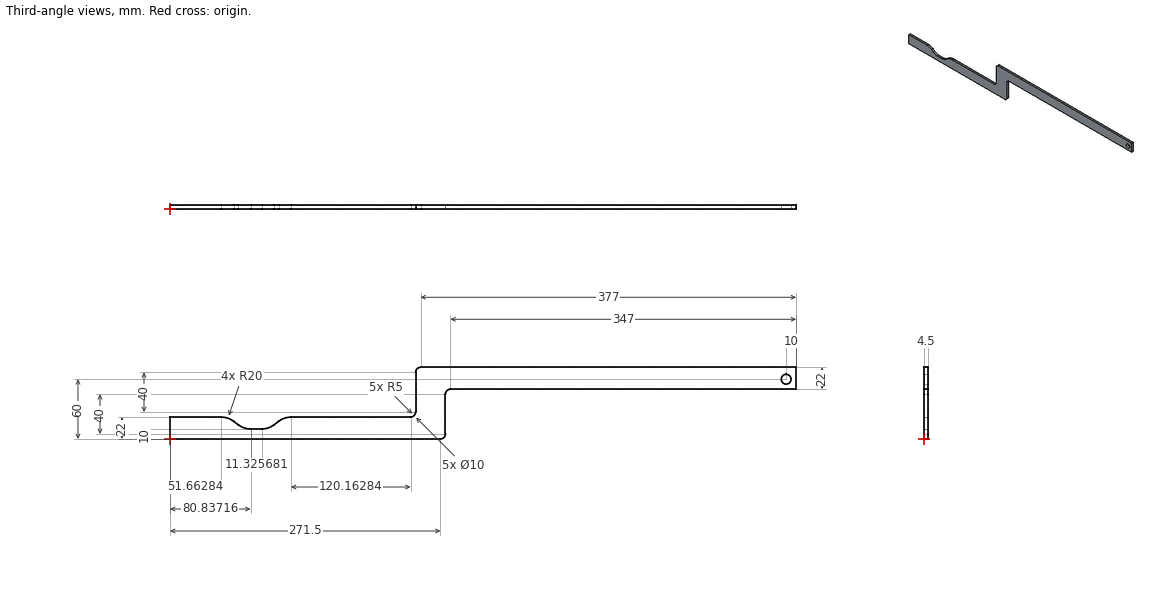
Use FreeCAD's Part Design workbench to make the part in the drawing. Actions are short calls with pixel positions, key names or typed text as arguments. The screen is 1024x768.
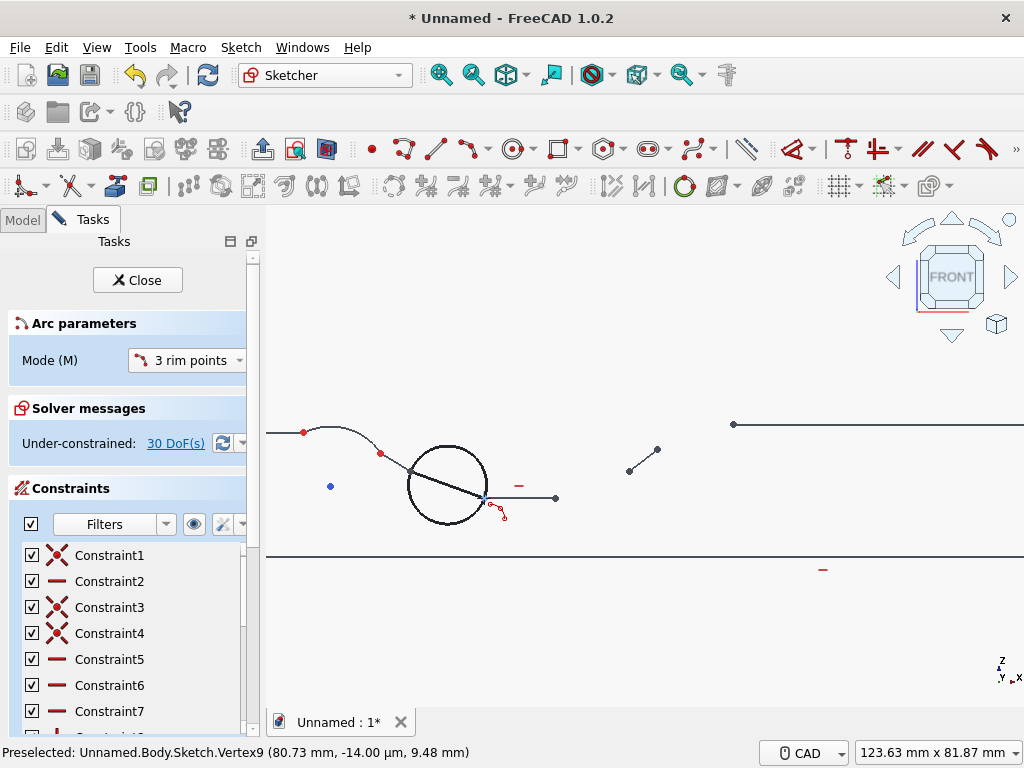
scroll(445, 489, up, 5)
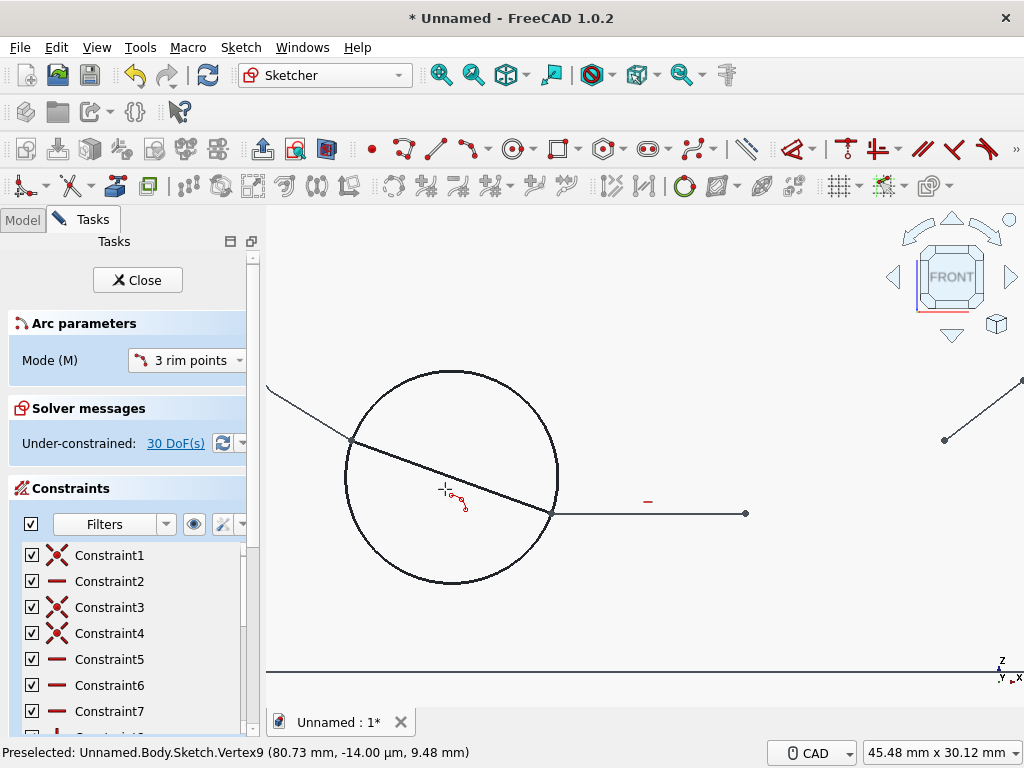
click(446, 487)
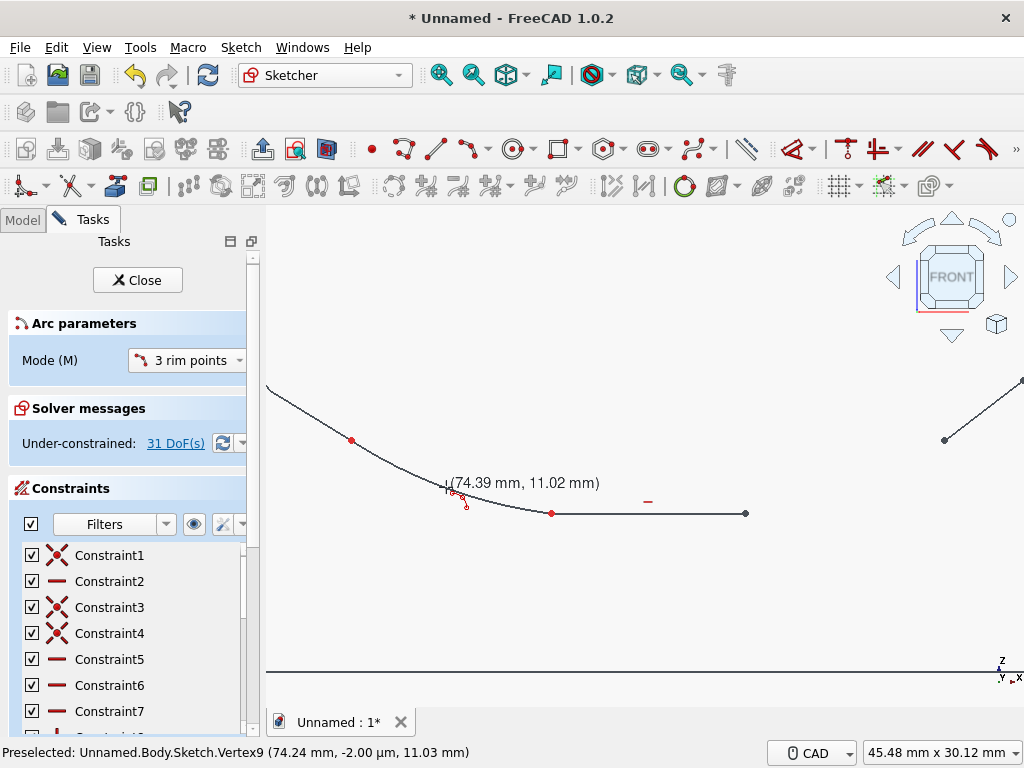
scroll(412, 472, down, 16)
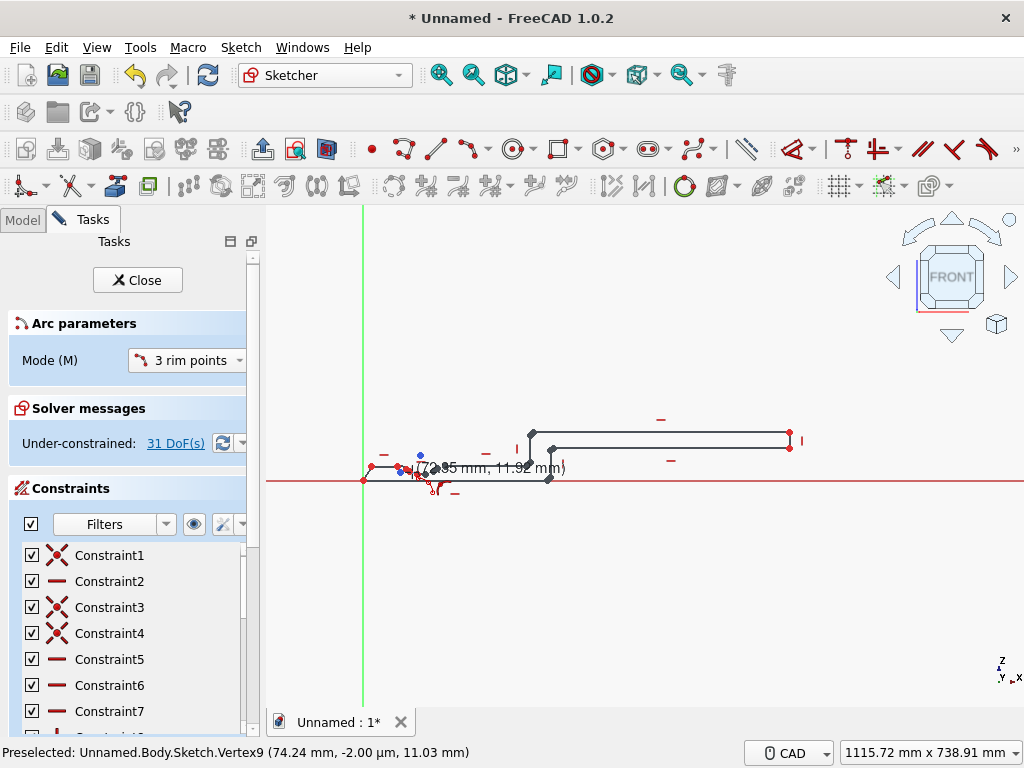
scroll(426, 474, up, 8)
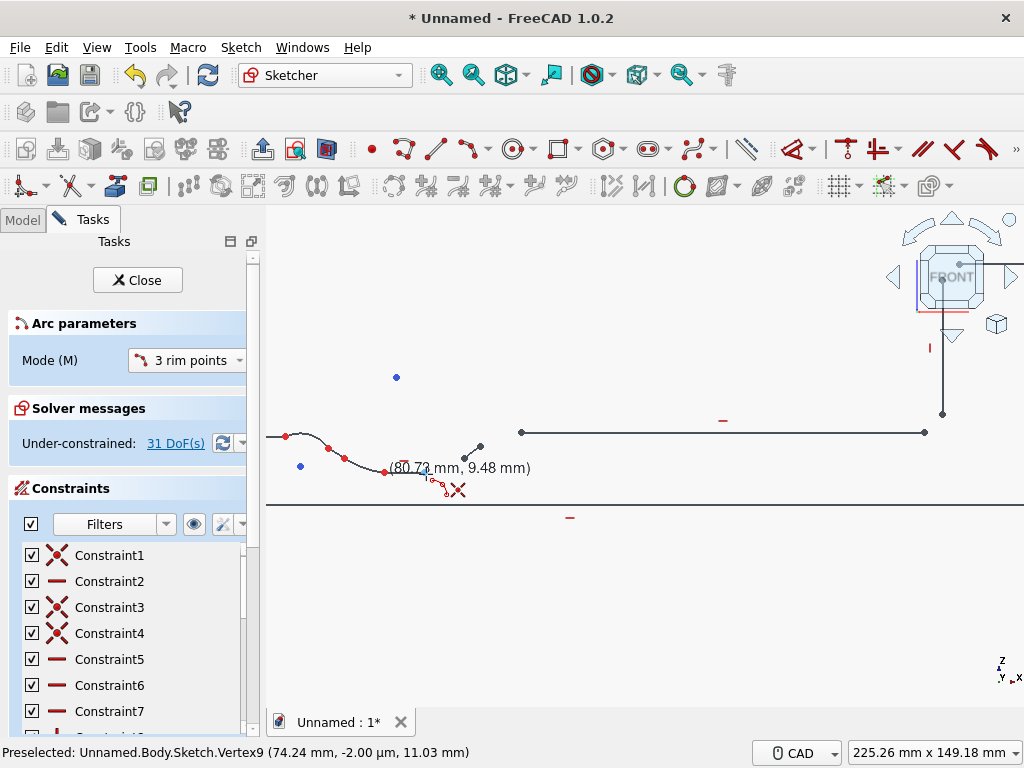
click(424, 473)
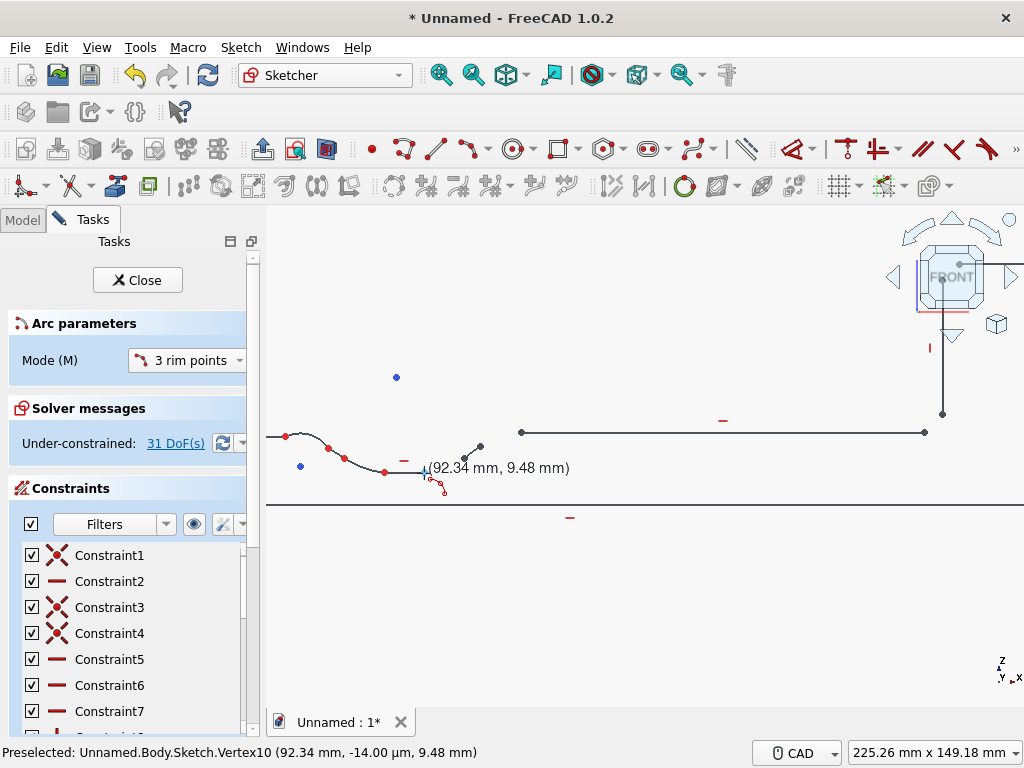
scroll(465, 457, up, 3)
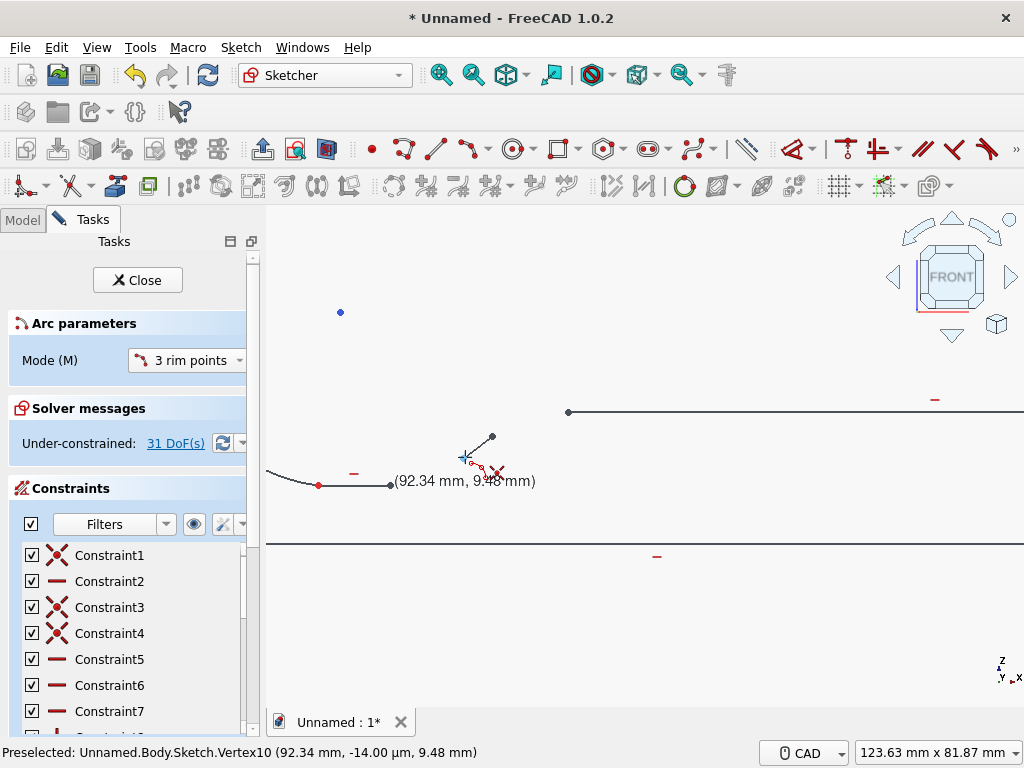
click(464, 459)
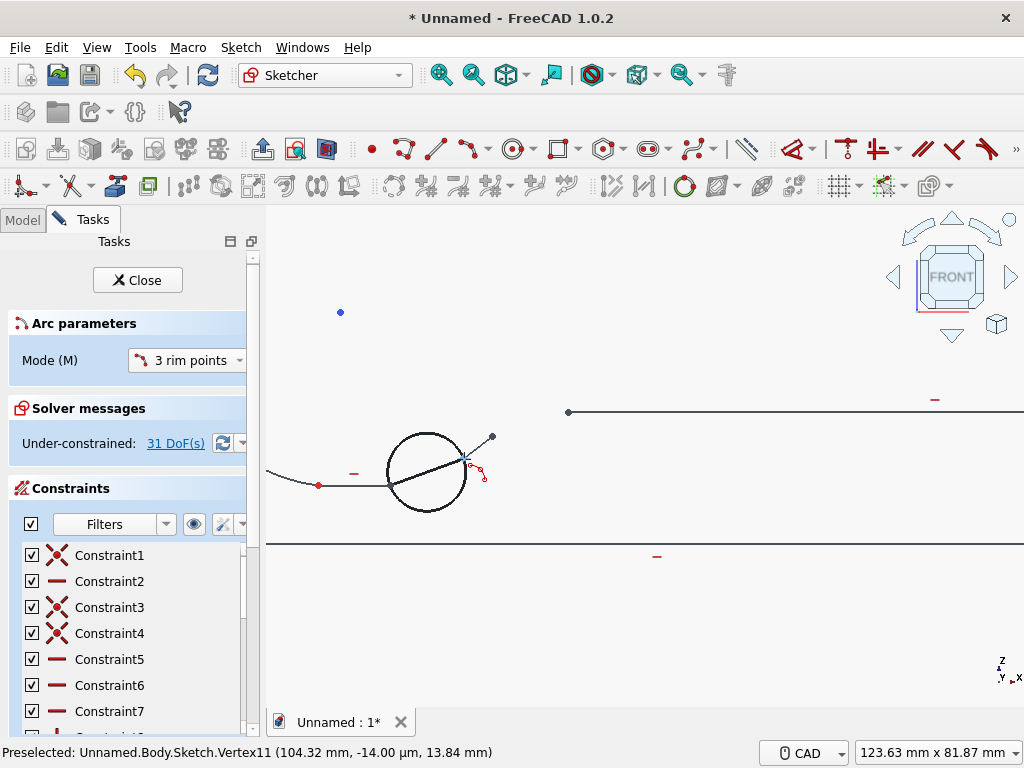
scroll(429, 476, up, 5)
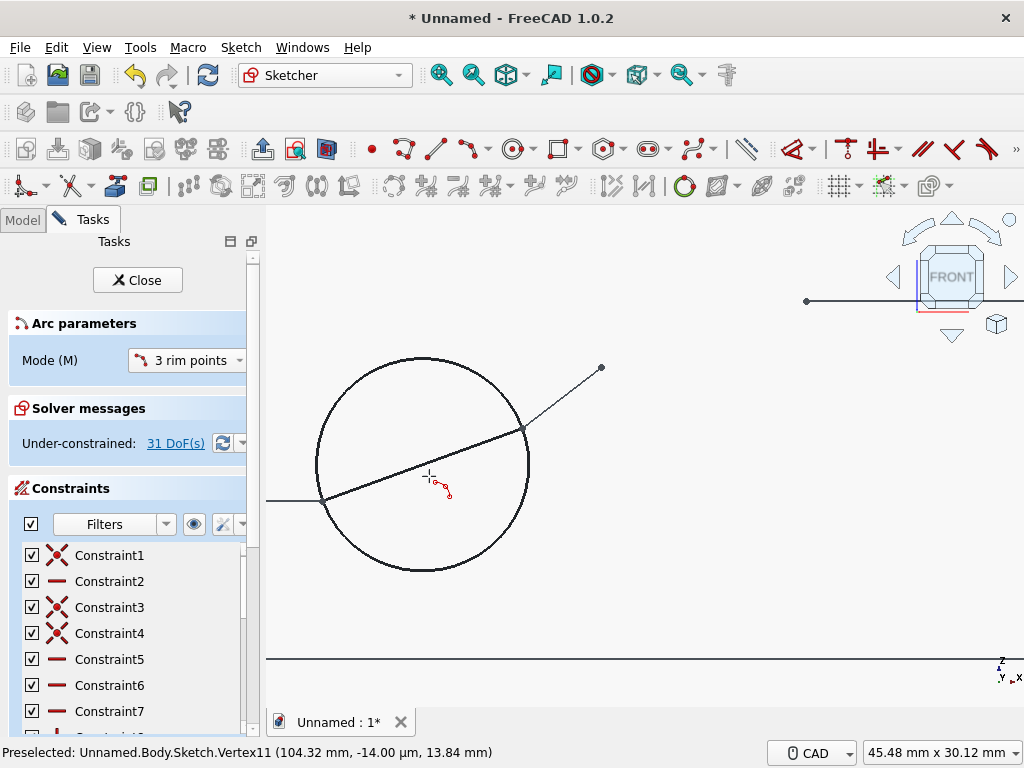
click(428, 474)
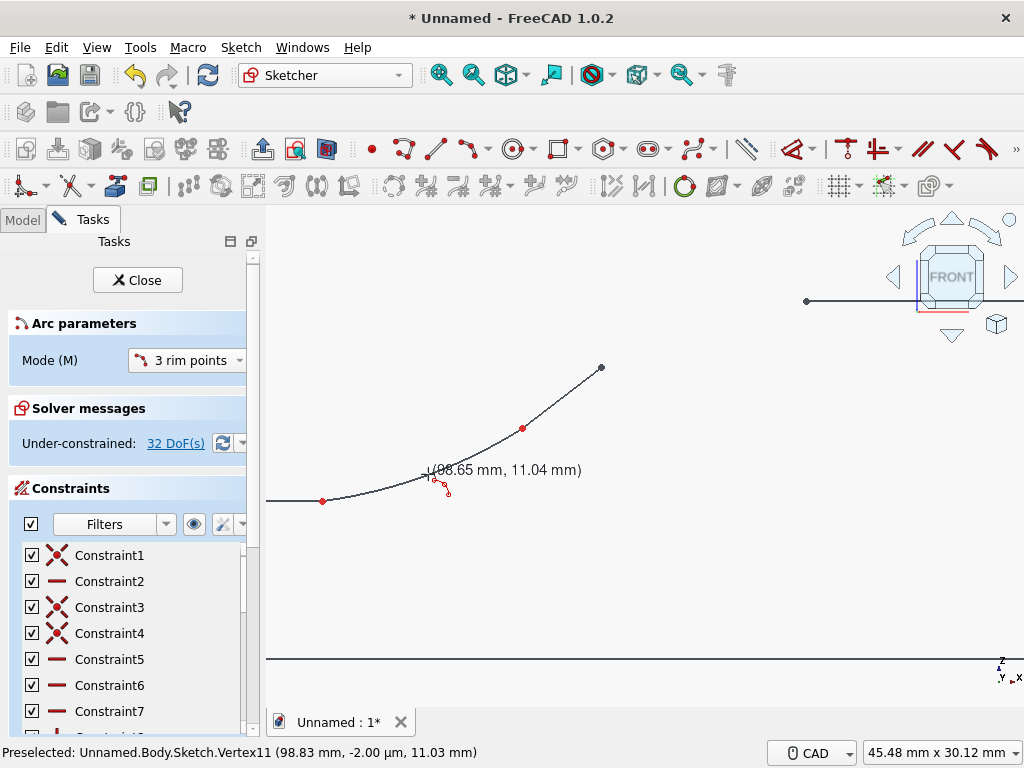
scroll(430, 473, down, 16)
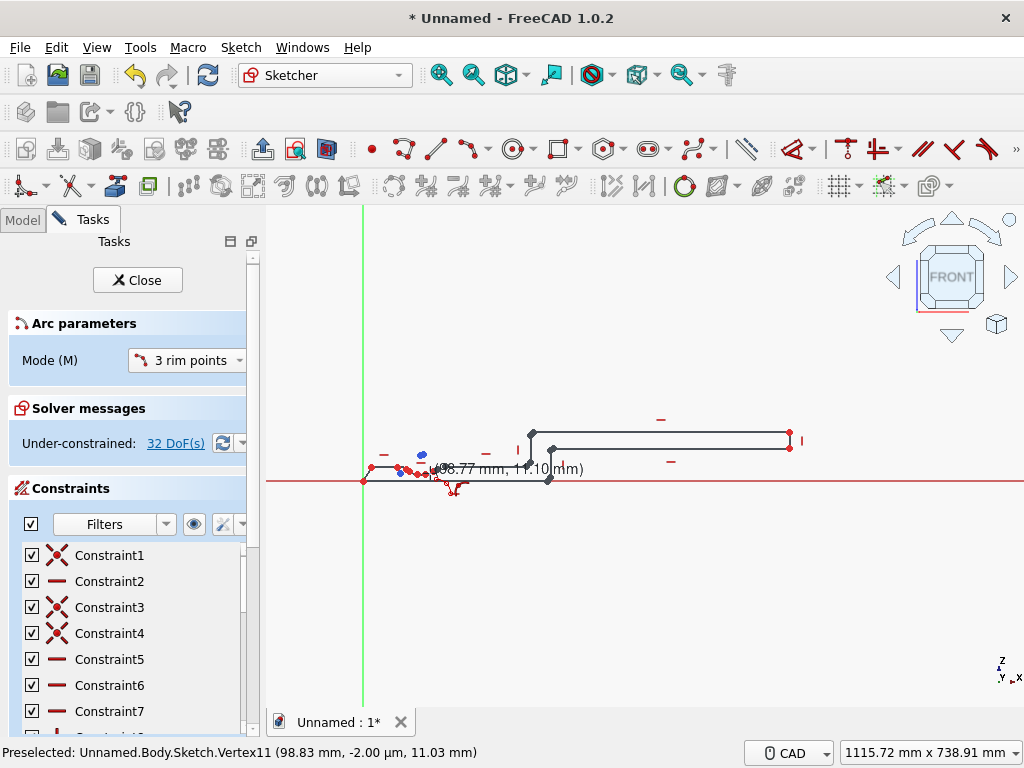
scroll(437, 469, up, 11)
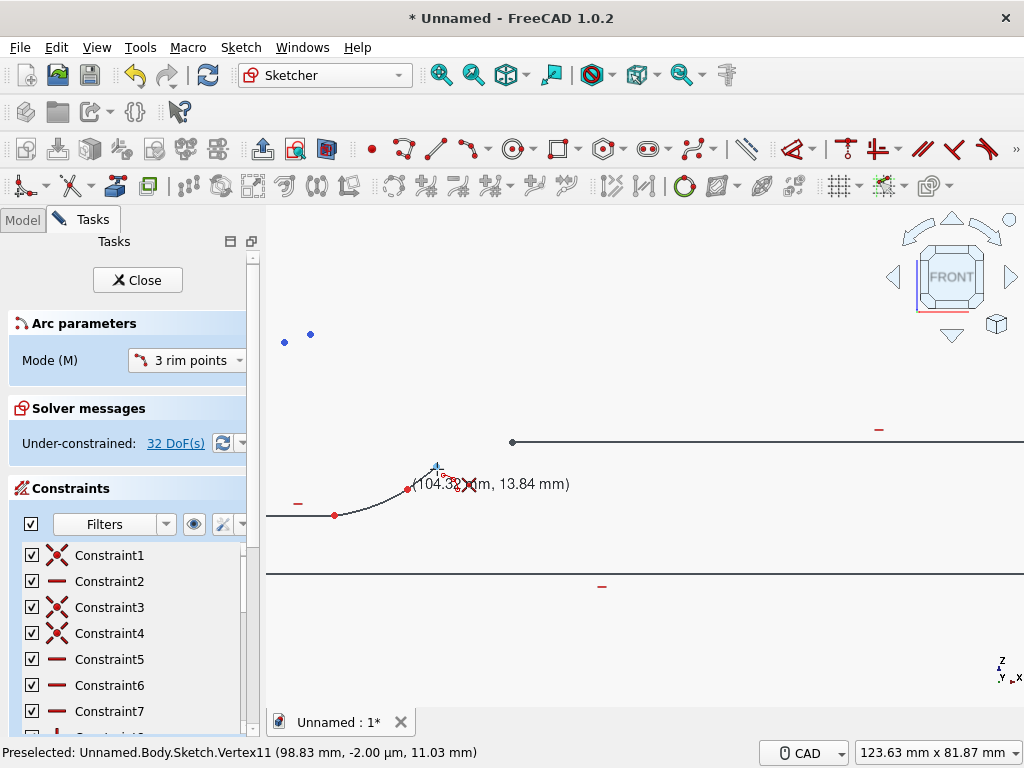
click(437, 467)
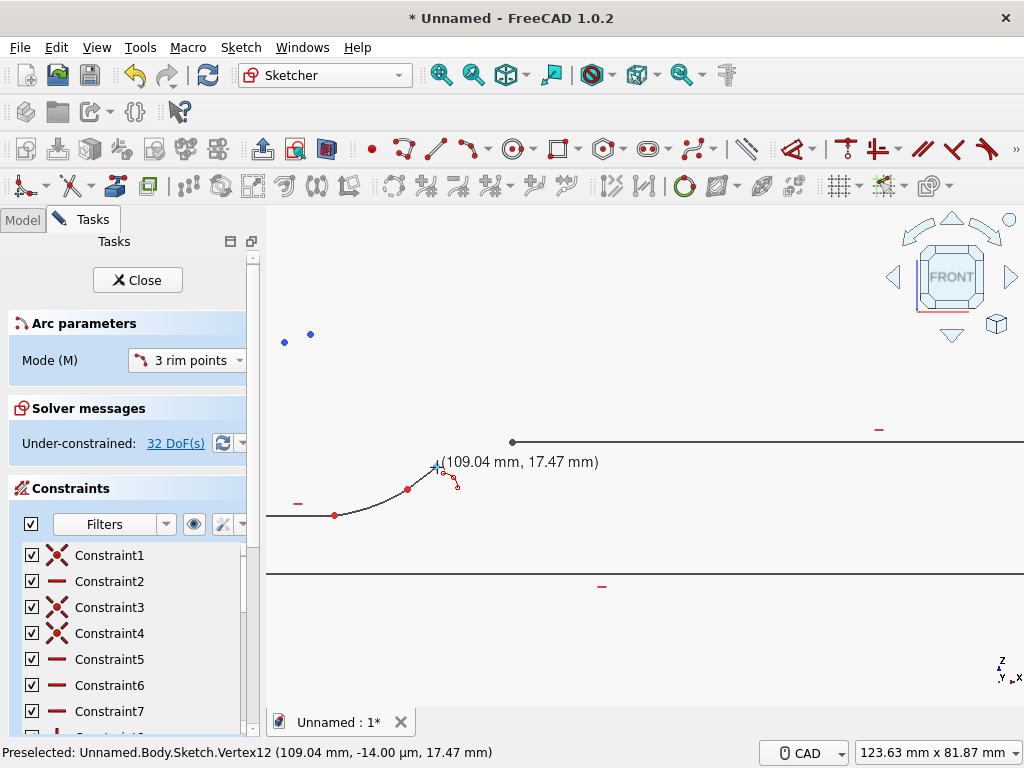
scroll(437, 469, down, 11)